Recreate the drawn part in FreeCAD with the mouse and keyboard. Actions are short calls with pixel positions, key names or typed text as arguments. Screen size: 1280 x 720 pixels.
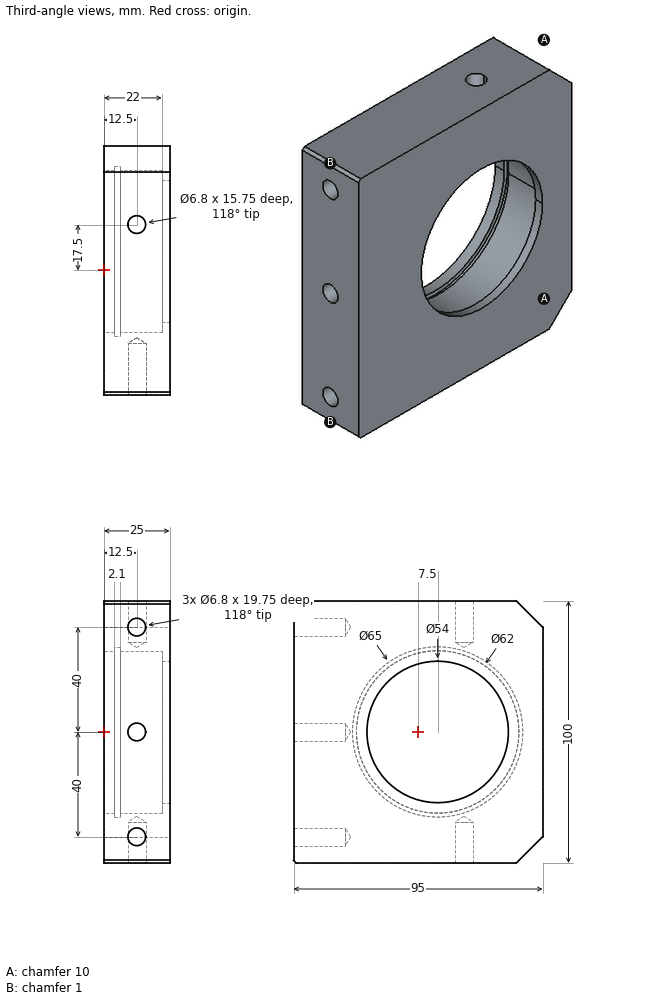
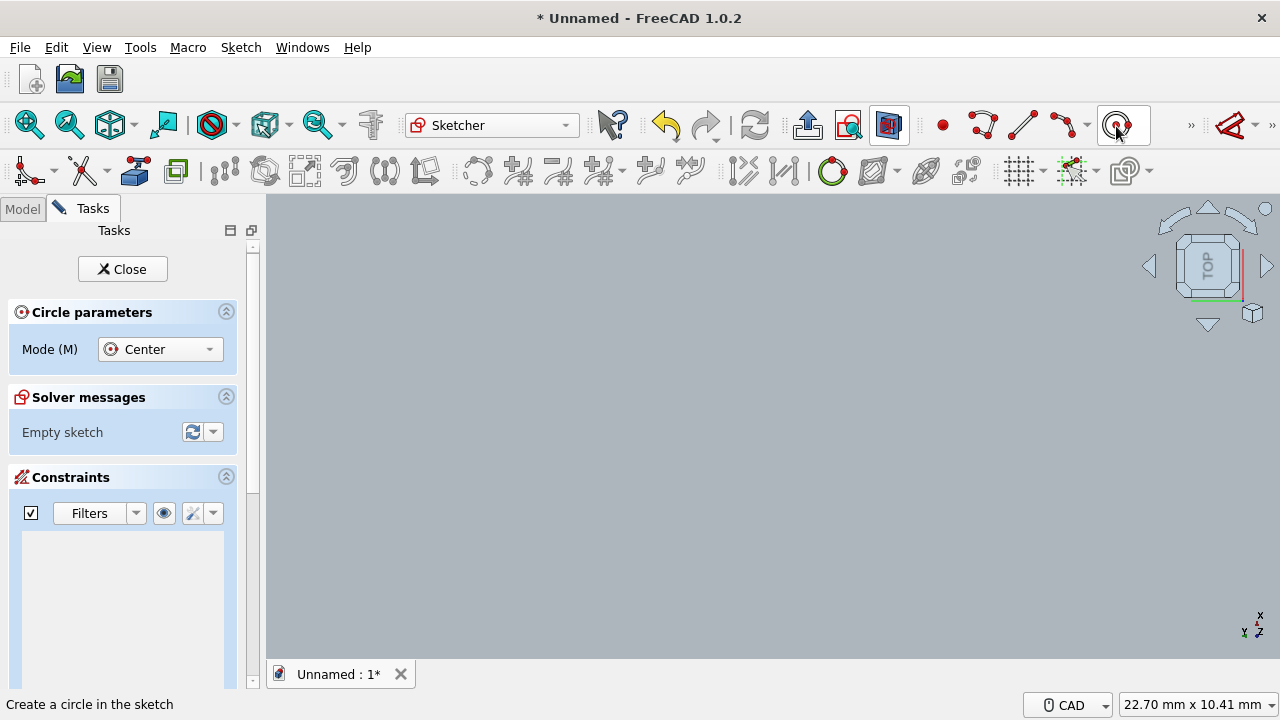
click(696, 414)
click(804, 307)
key(Escape)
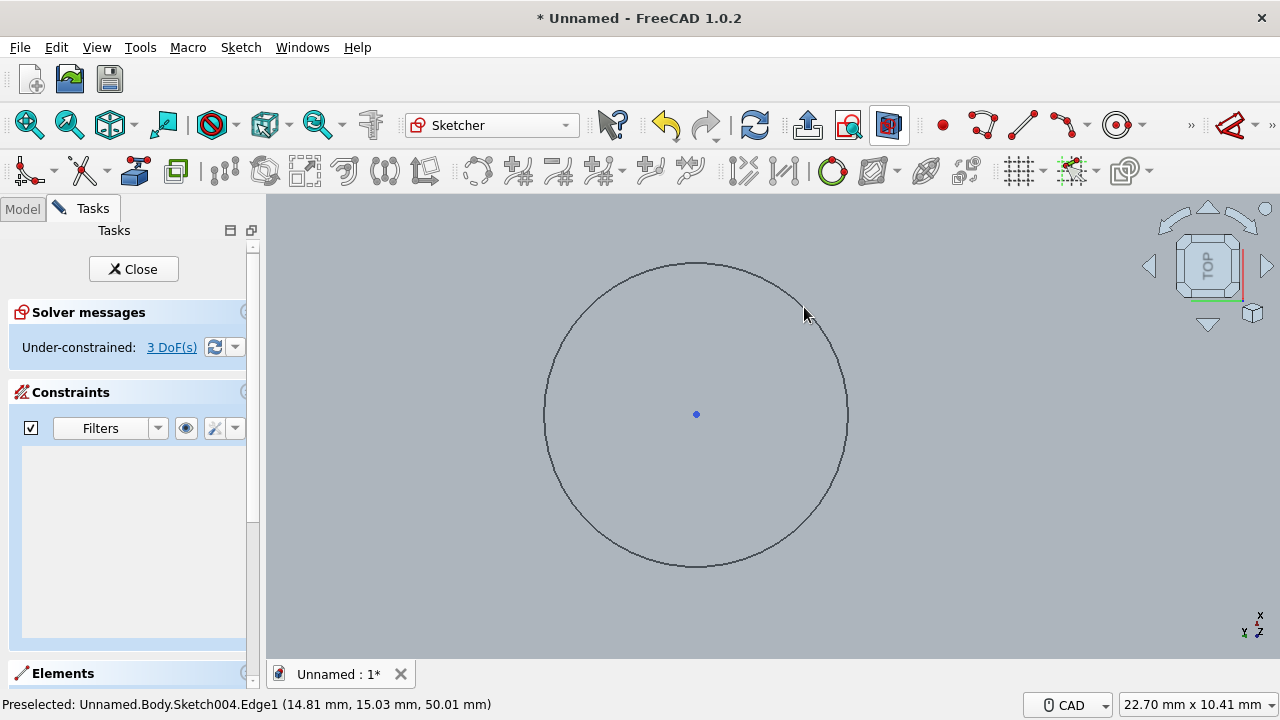
click(1230, 126)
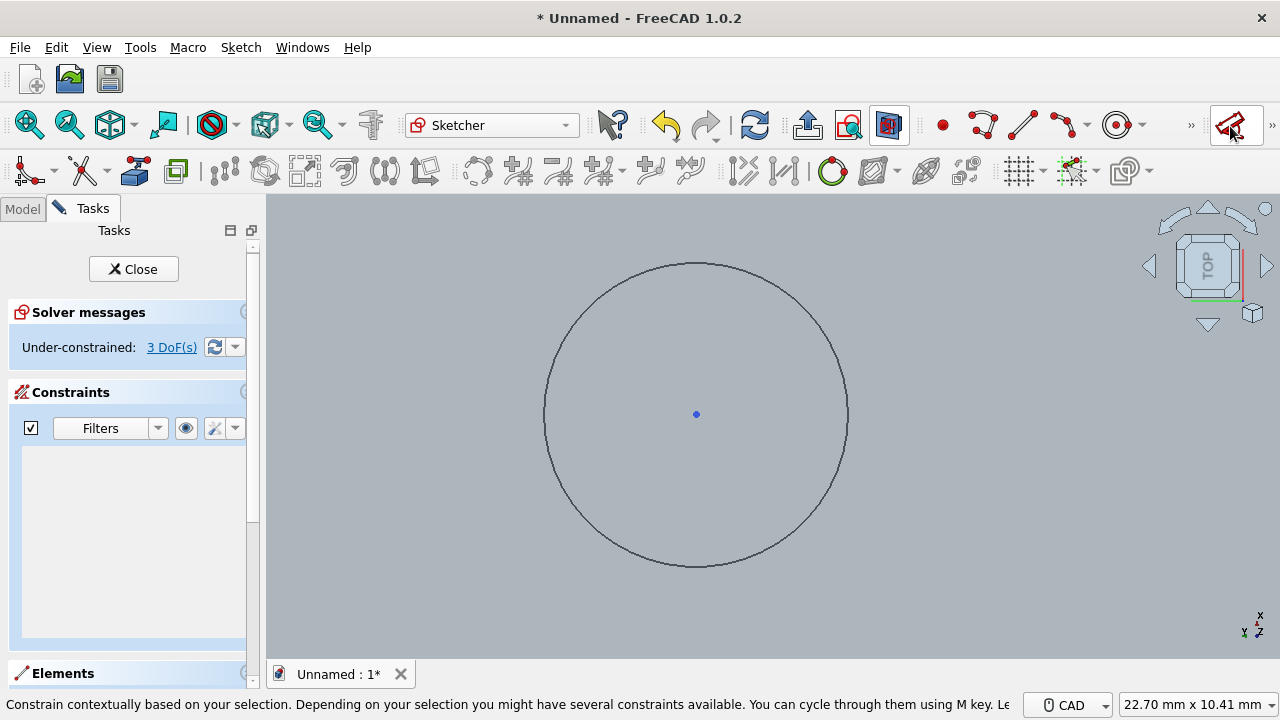
click(803, 307)
click(826, 284)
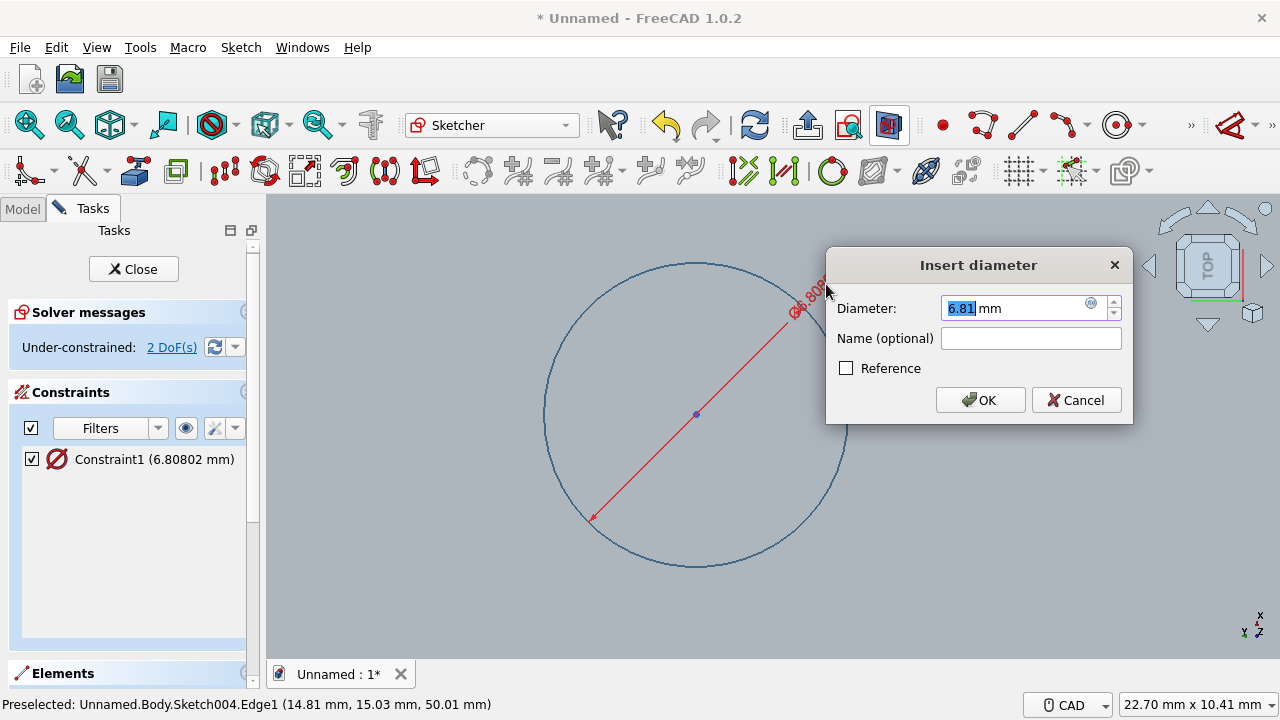
text(6.8)
key(Return)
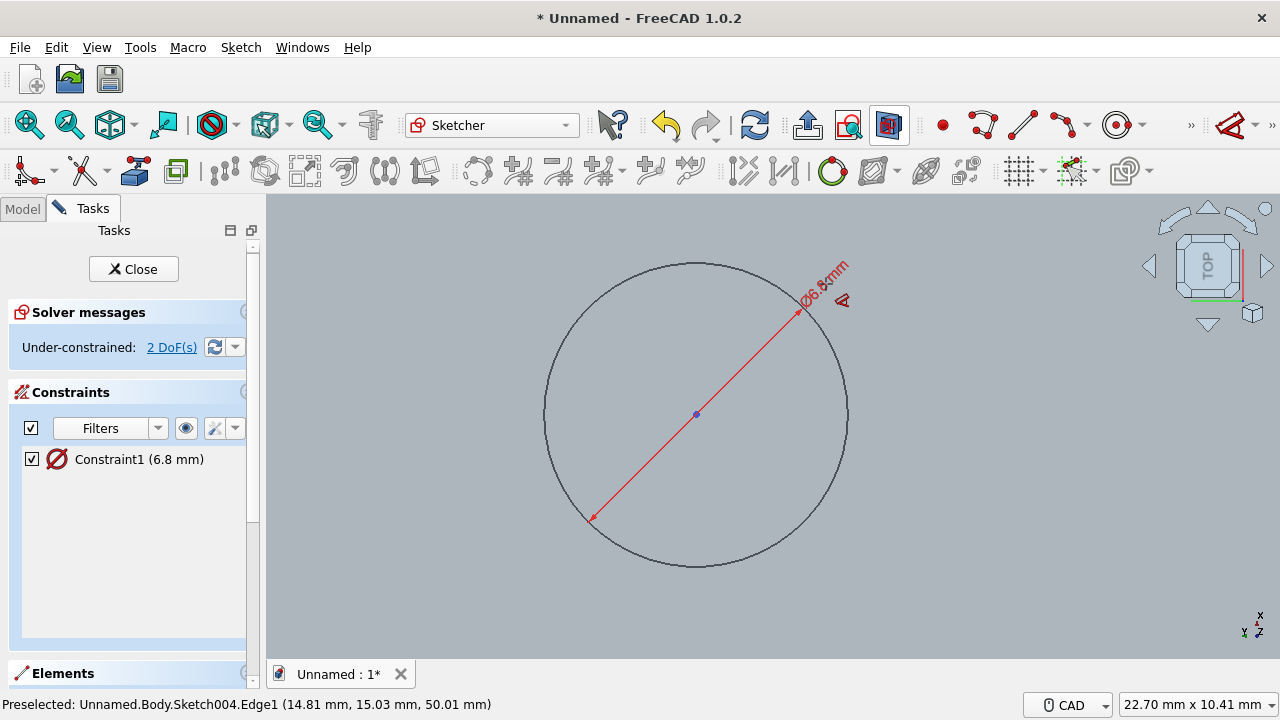
click(696, 415)
click(906, 381)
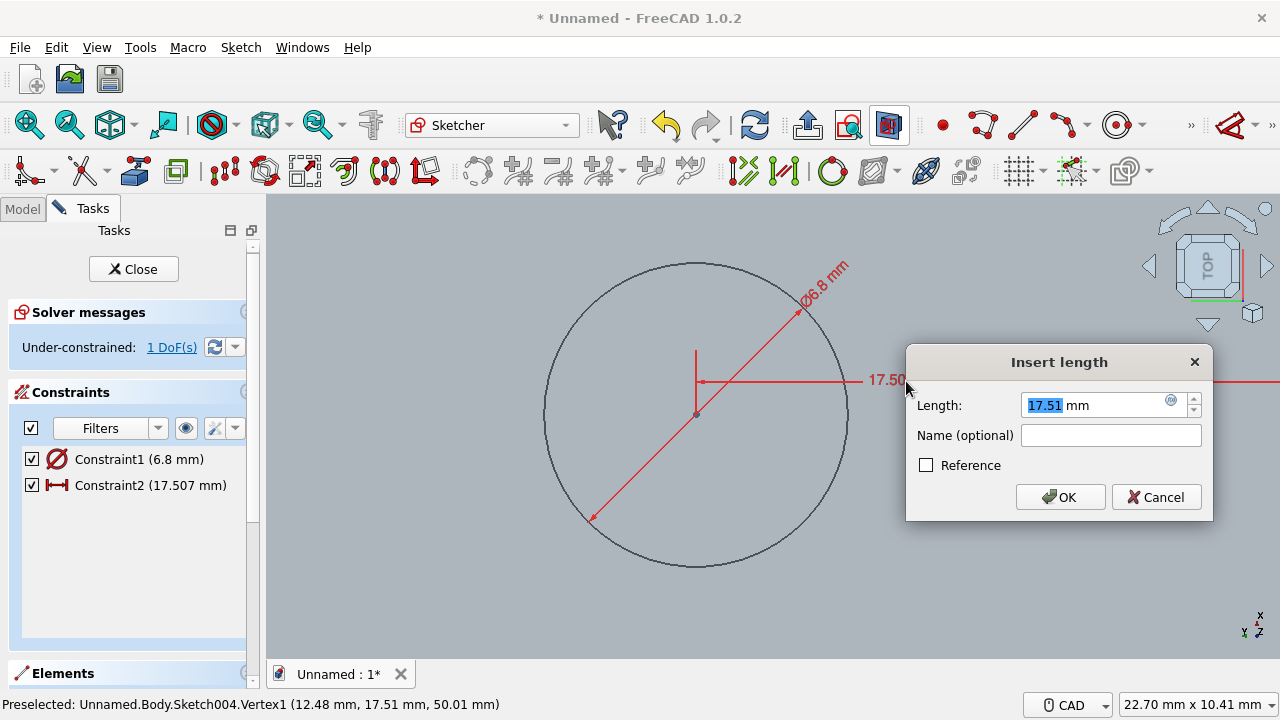
text(17.5)
key(Return)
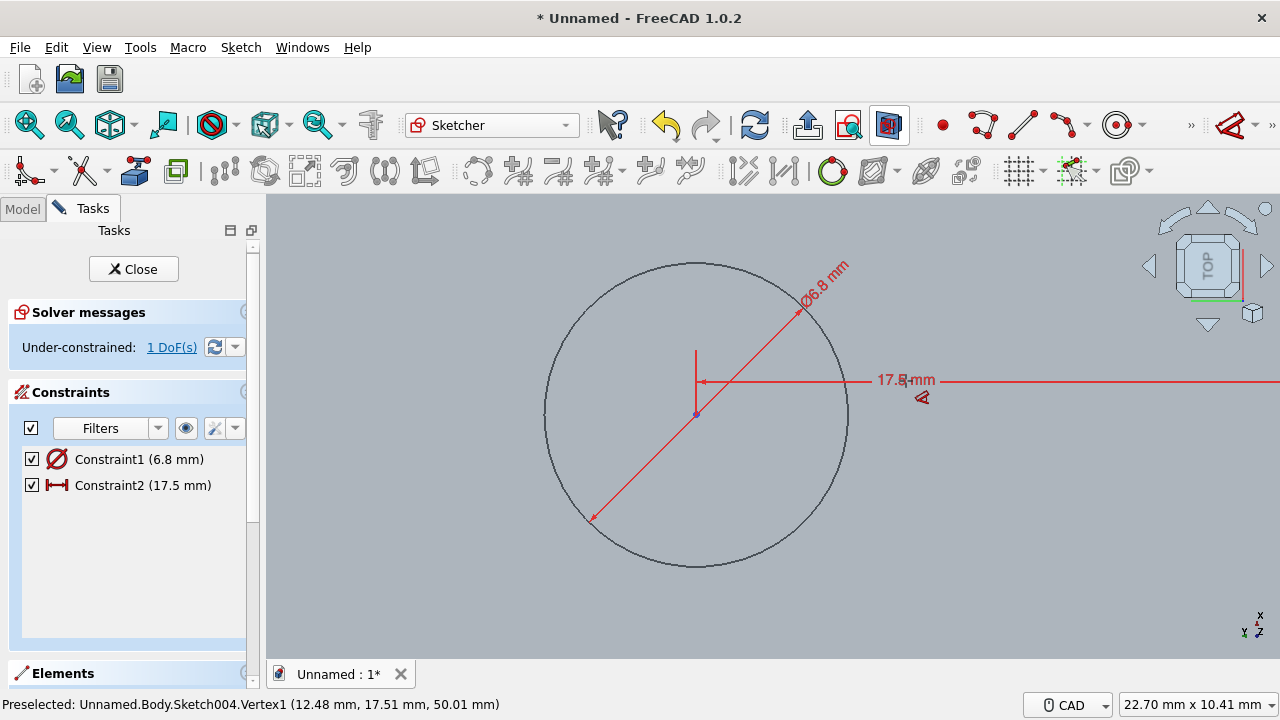
click(696, 415)
click(662, 523)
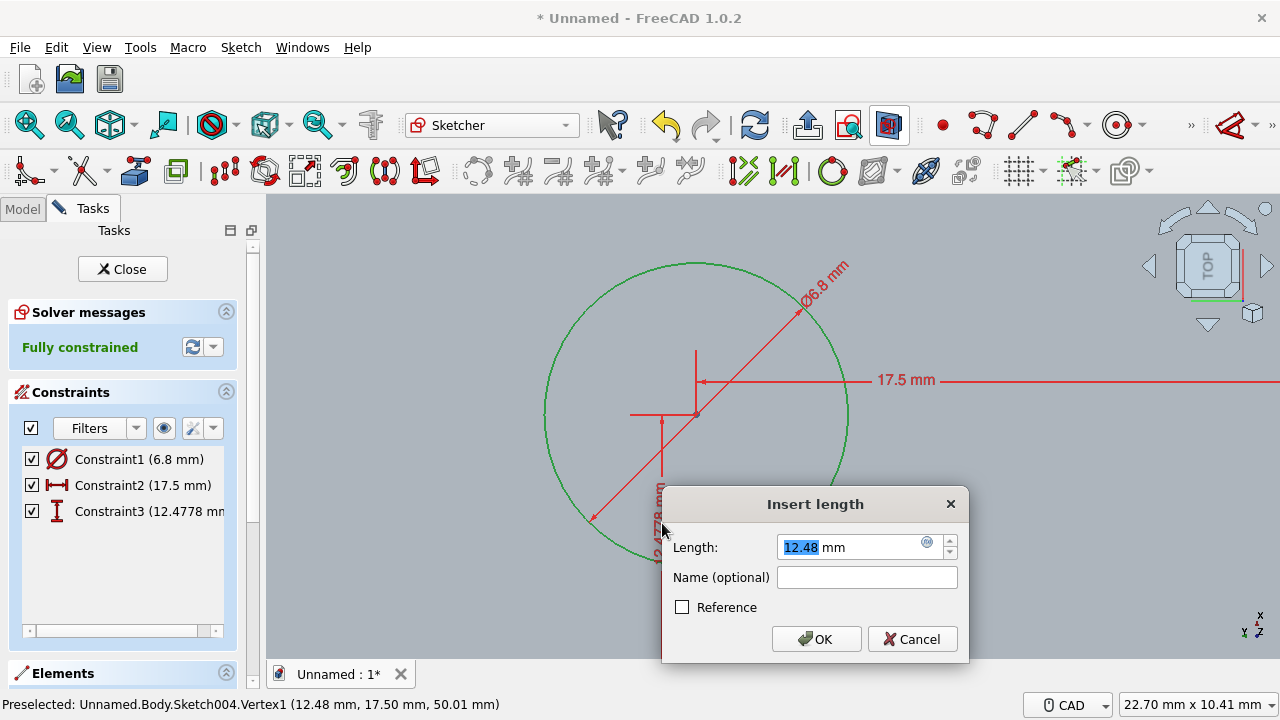
text(12.5)
key(Return)
key(Escape)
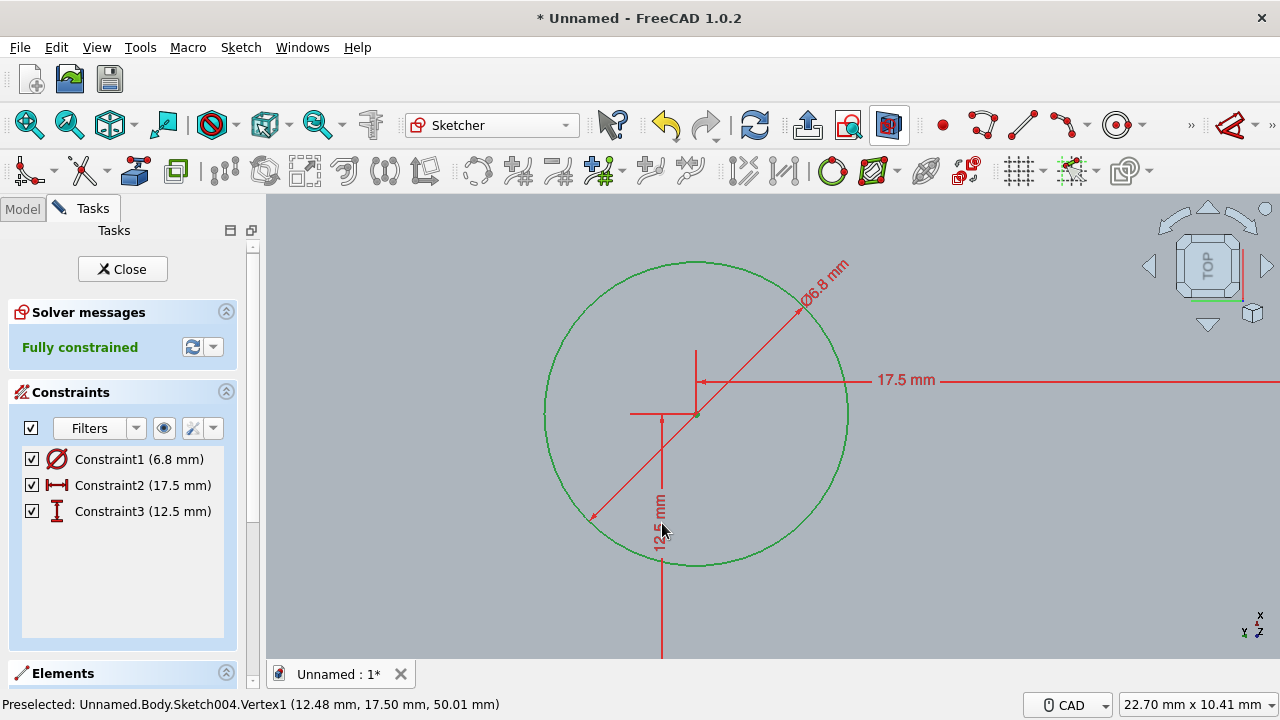
click(123, 269)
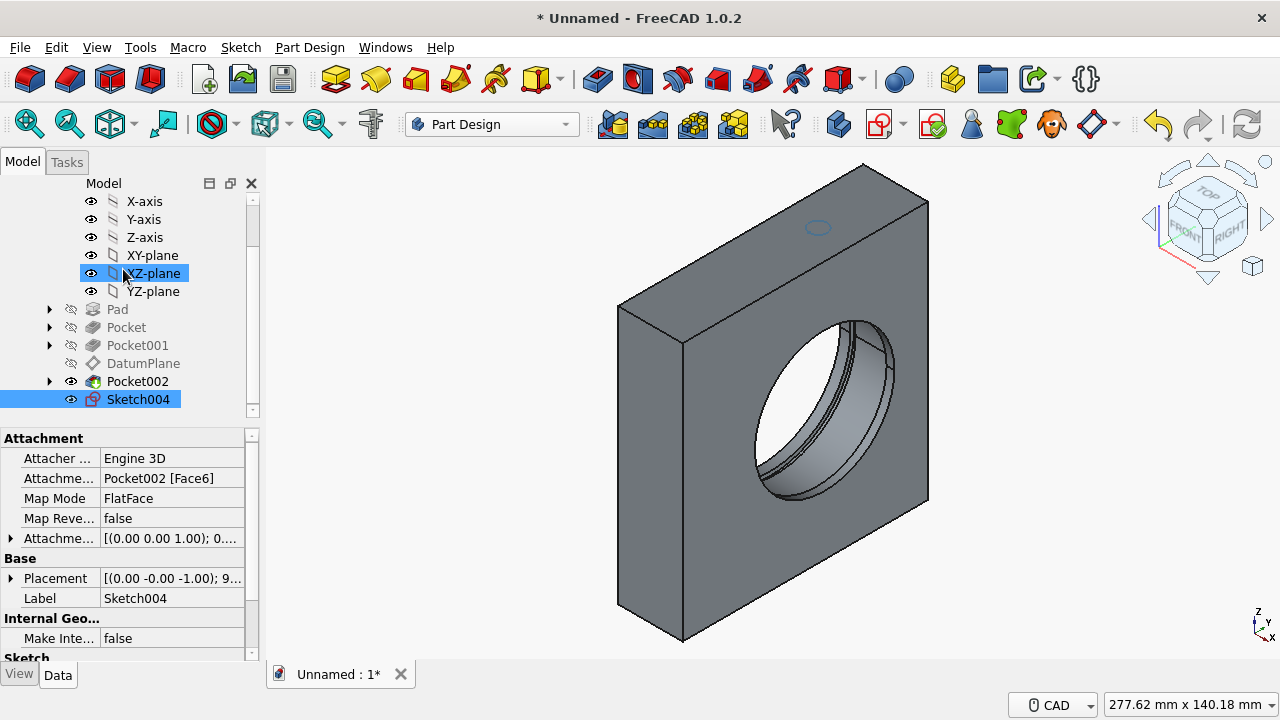
click(638, 80)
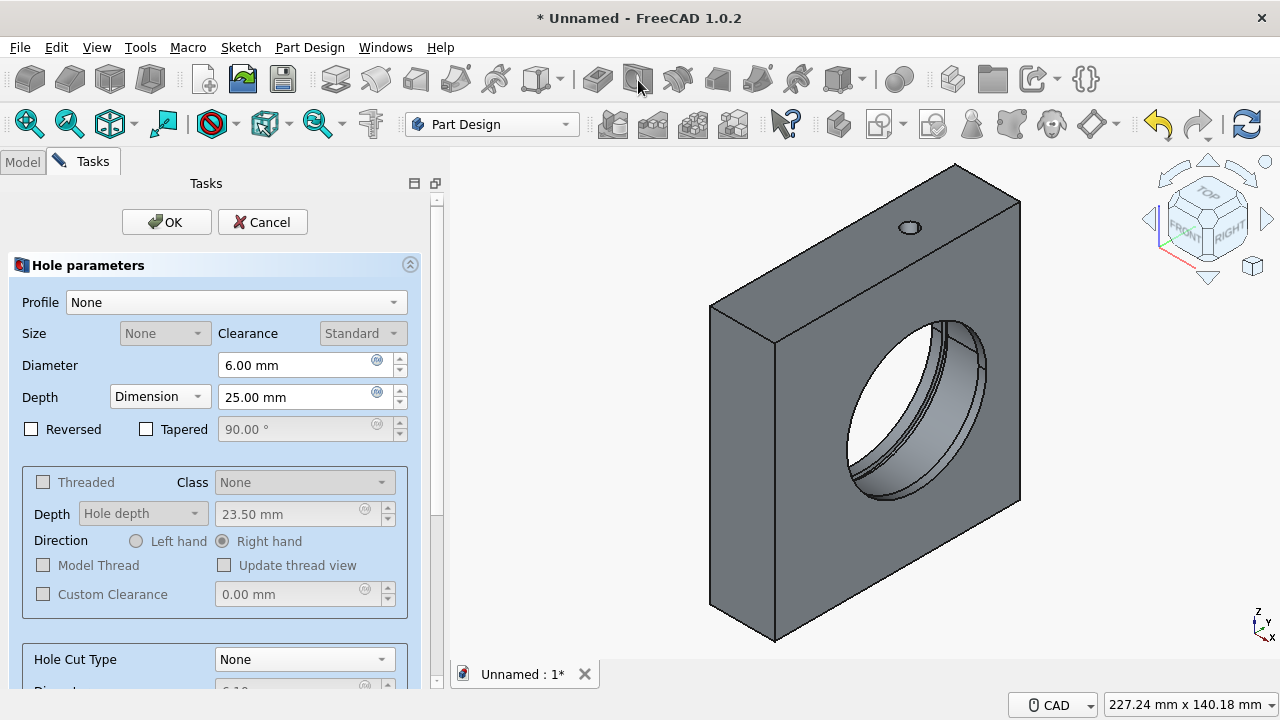
triple_click(305, 365)